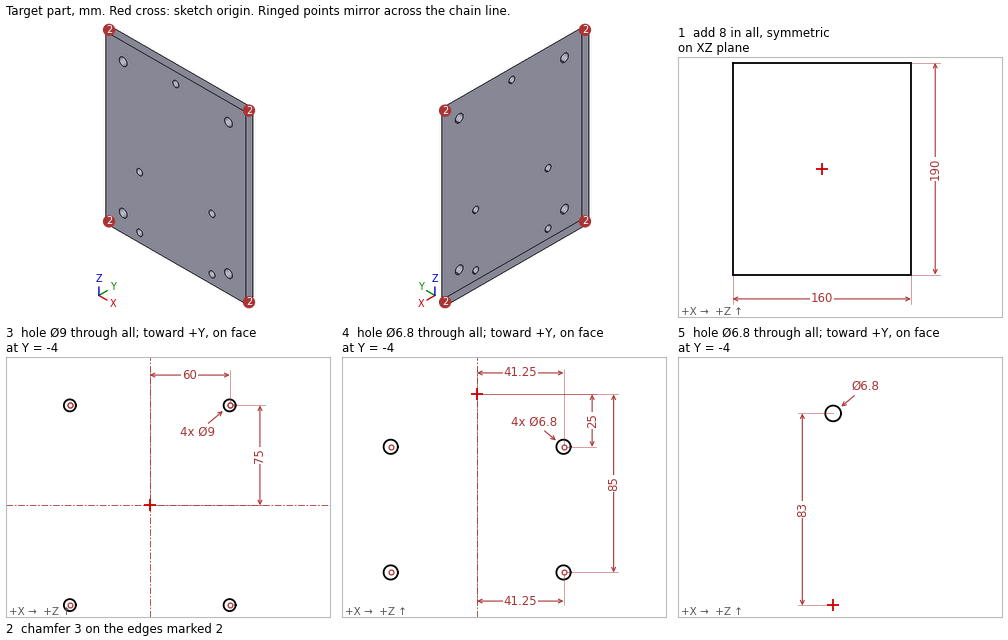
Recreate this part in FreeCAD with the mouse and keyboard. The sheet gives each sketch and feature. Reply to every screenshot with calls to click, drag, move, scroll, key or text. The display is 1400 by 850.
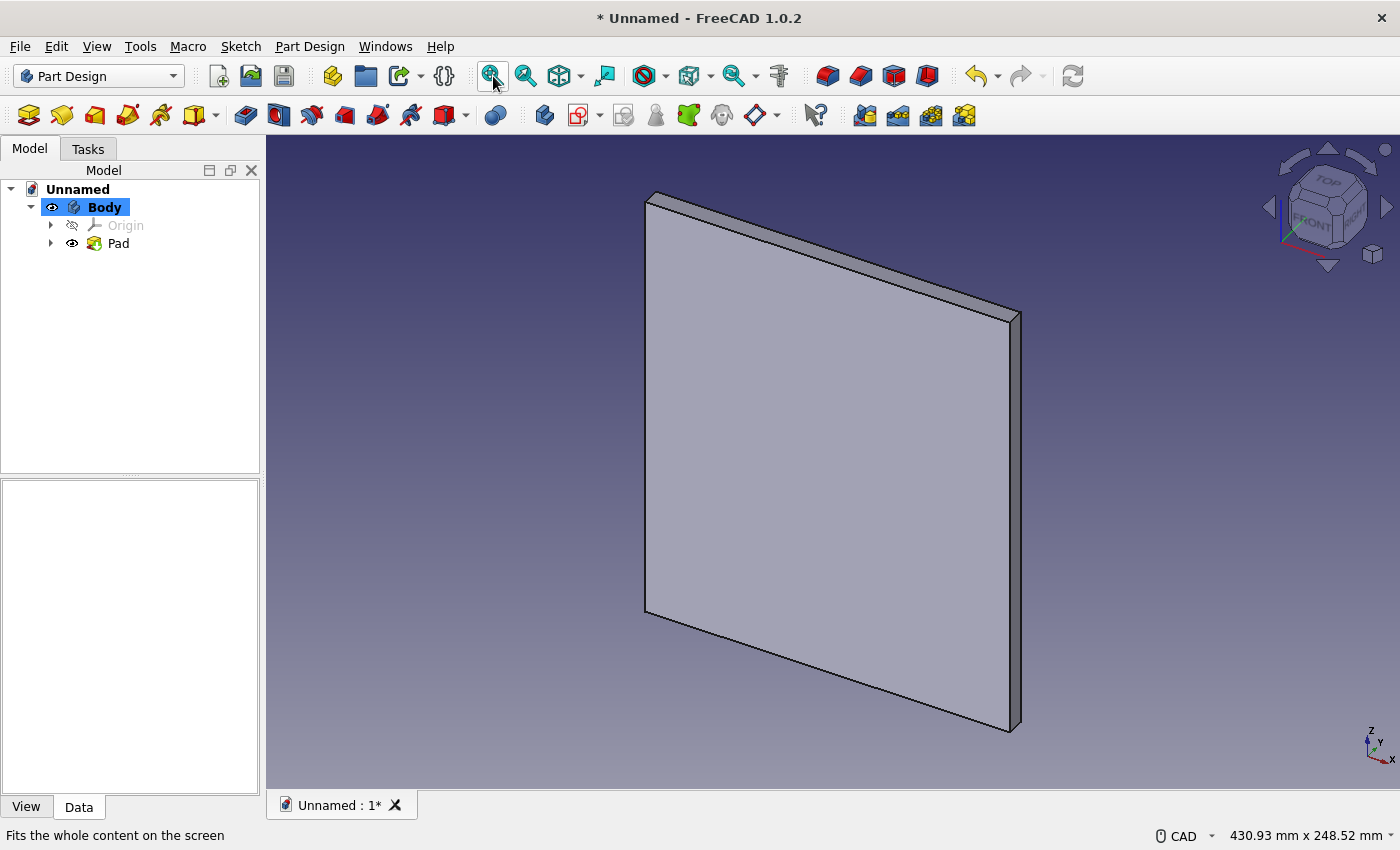
click(1015, 317)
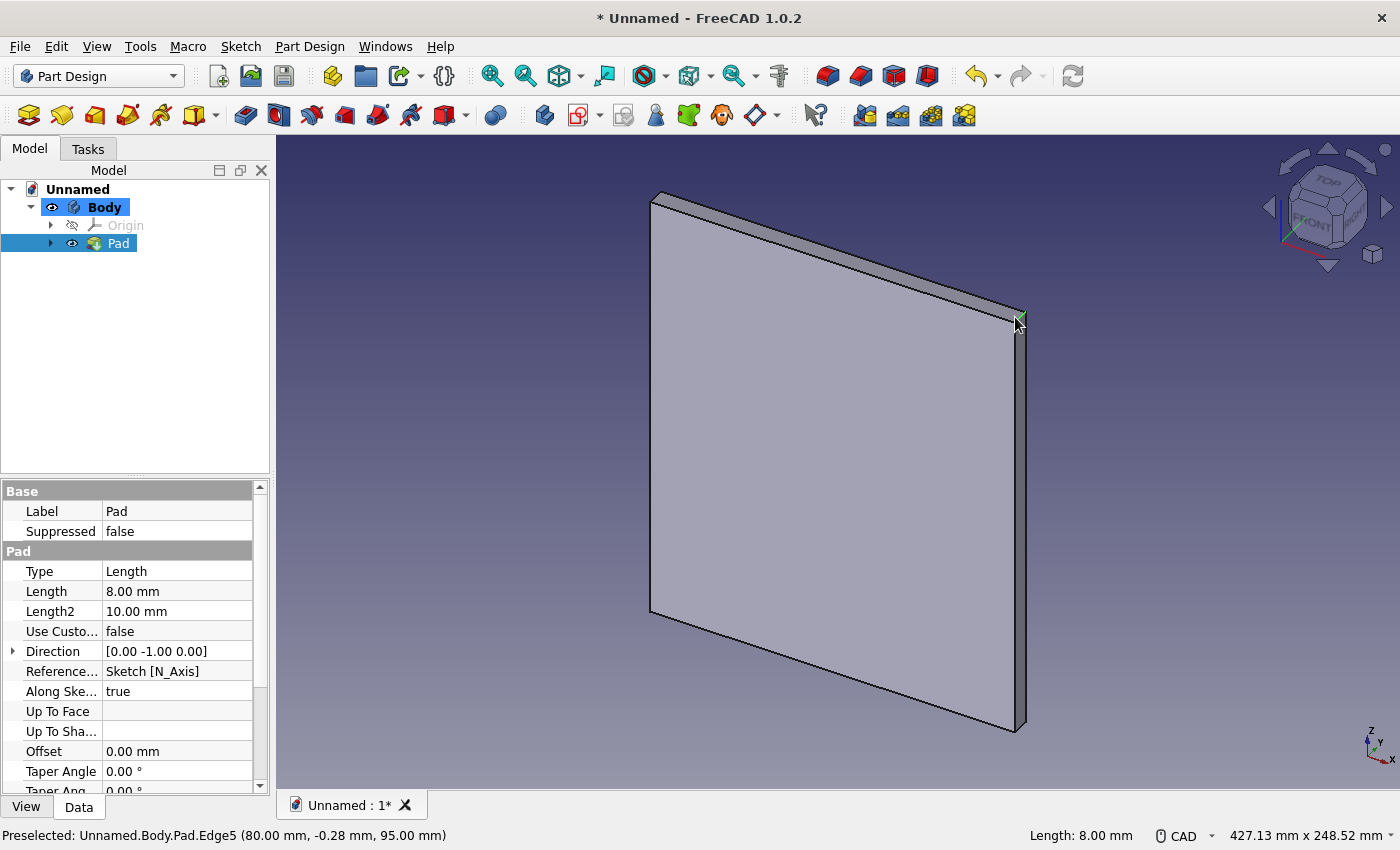
scroll(656, 196, up, 4)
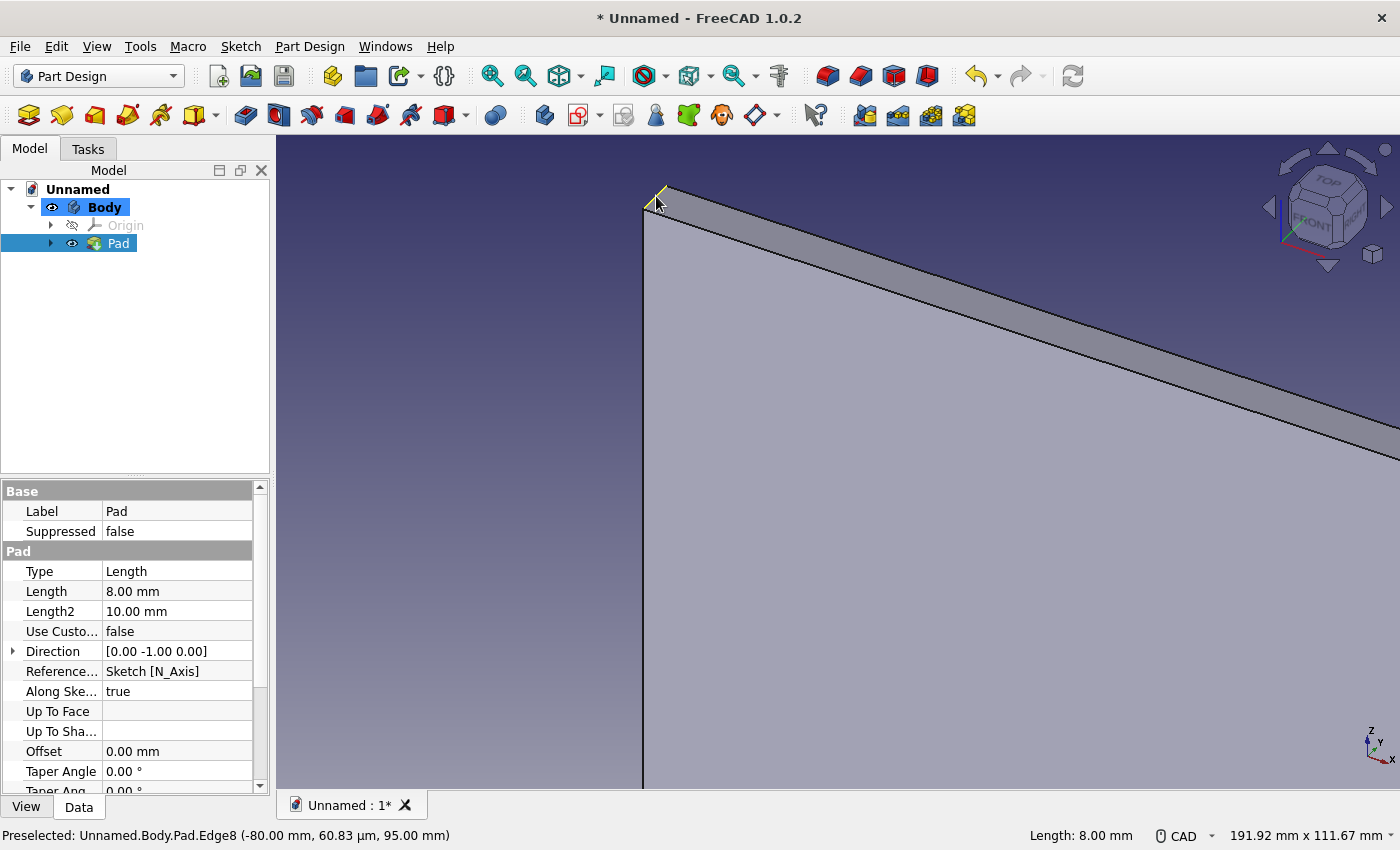
click(493, 76)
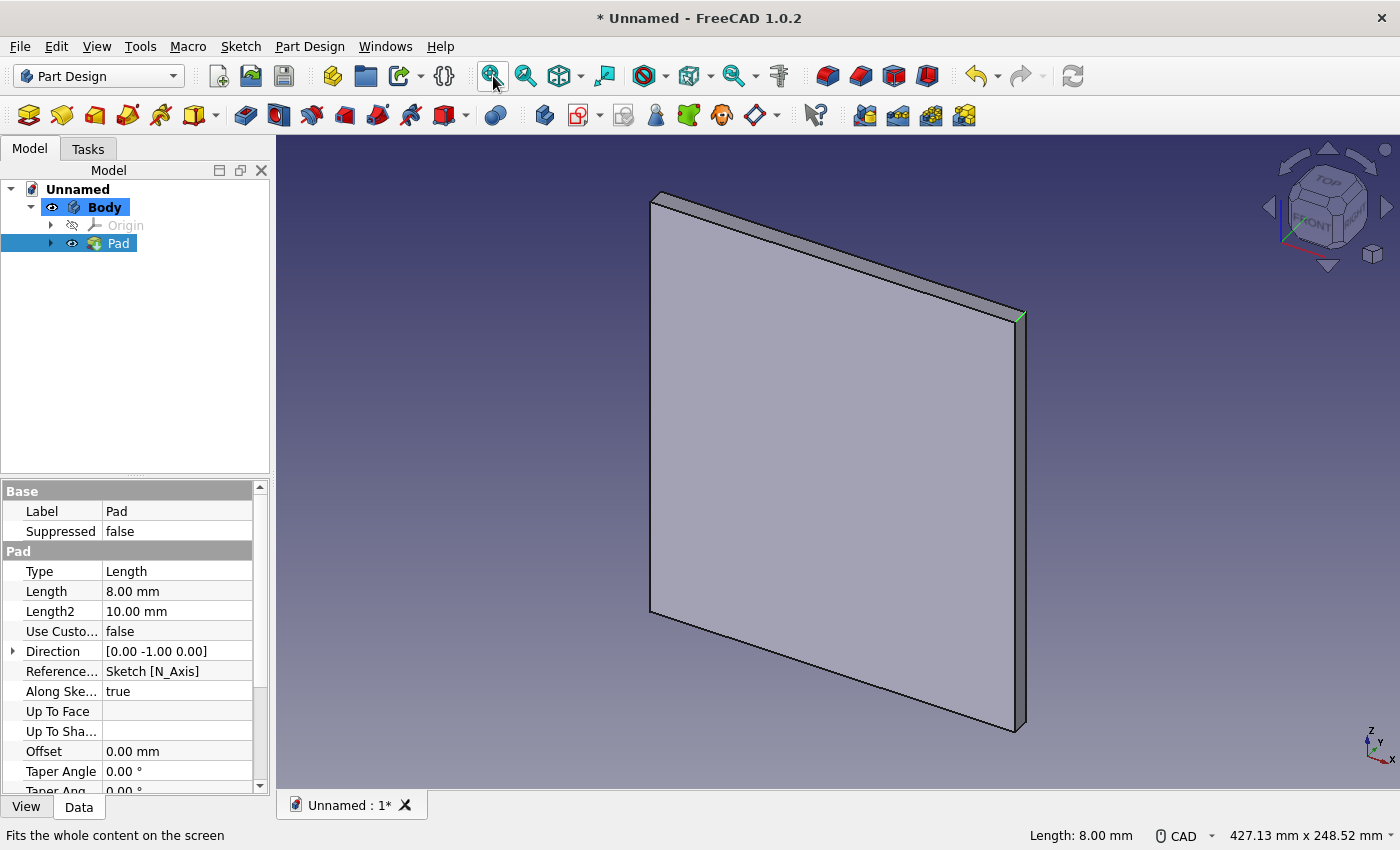
key(0)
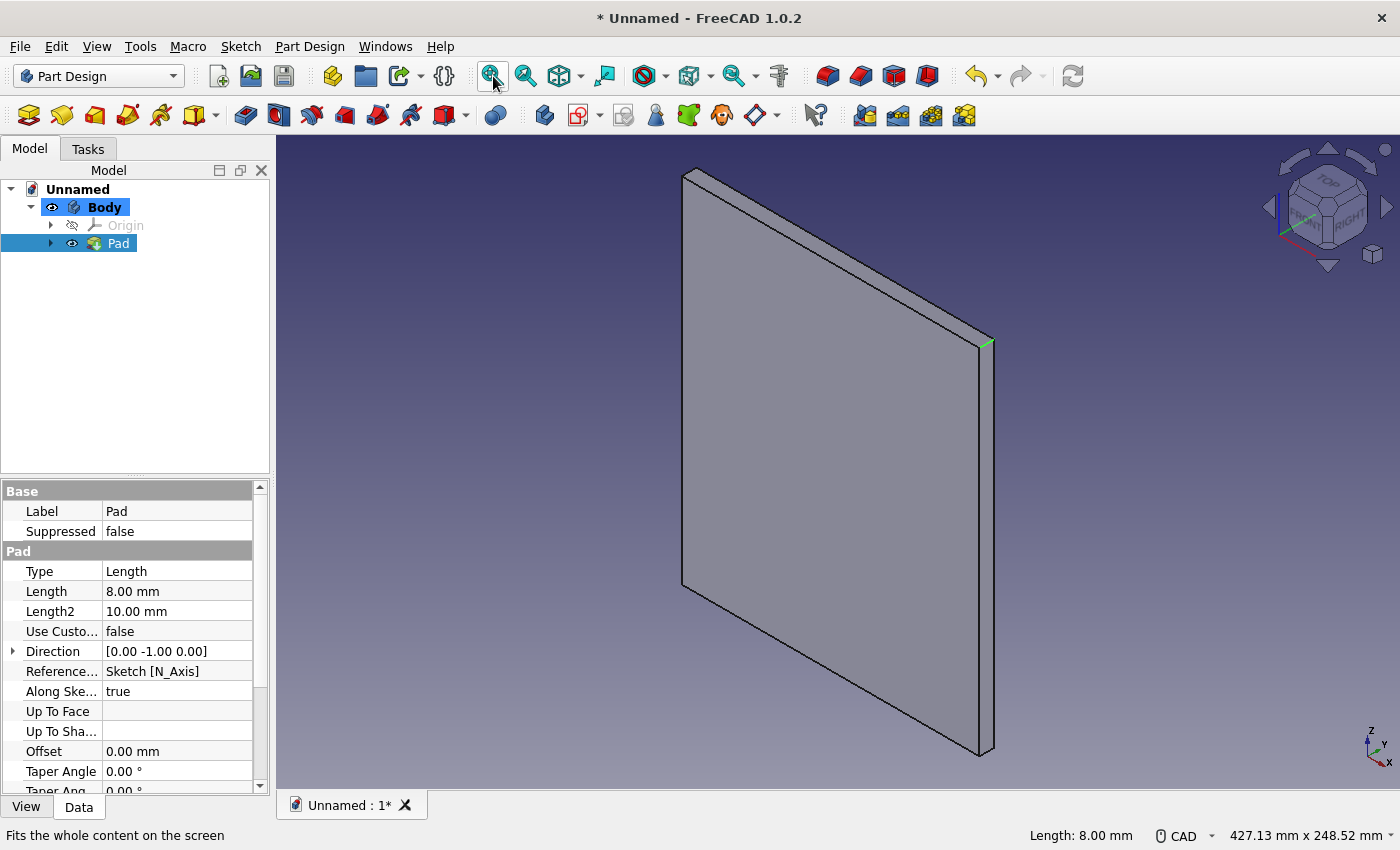
scroll(689, 171, up, 4)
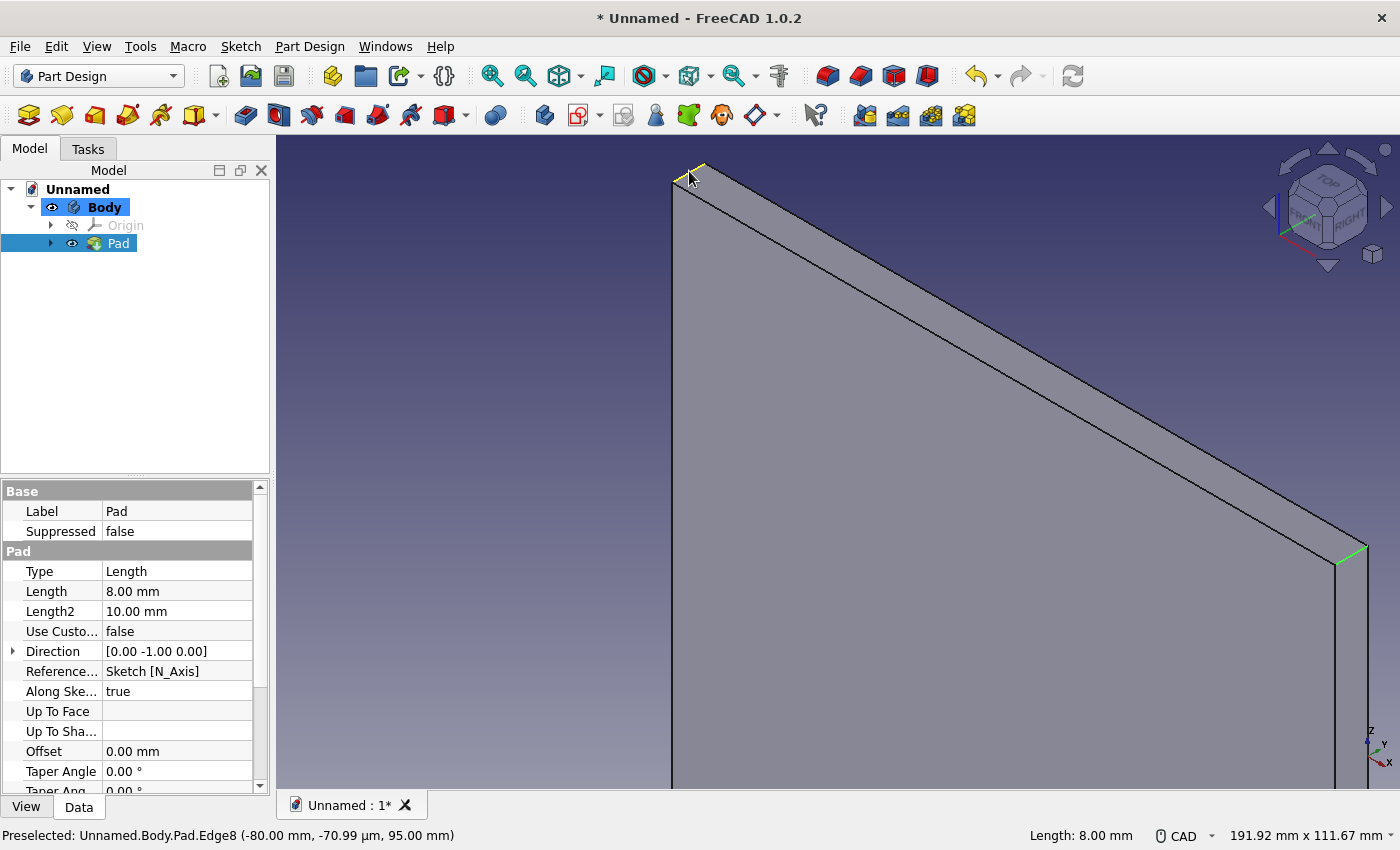
click(493, 76)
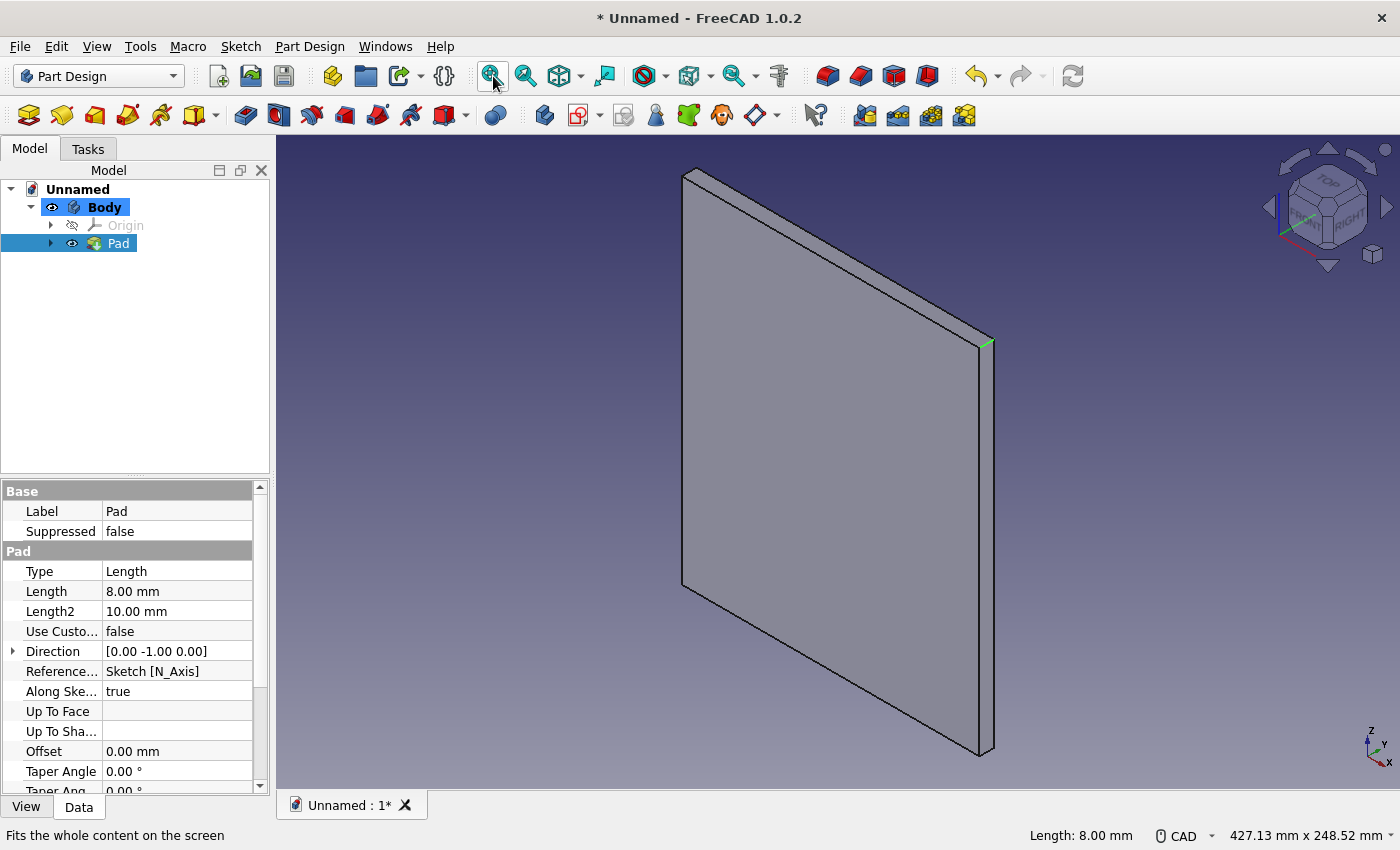
key(2)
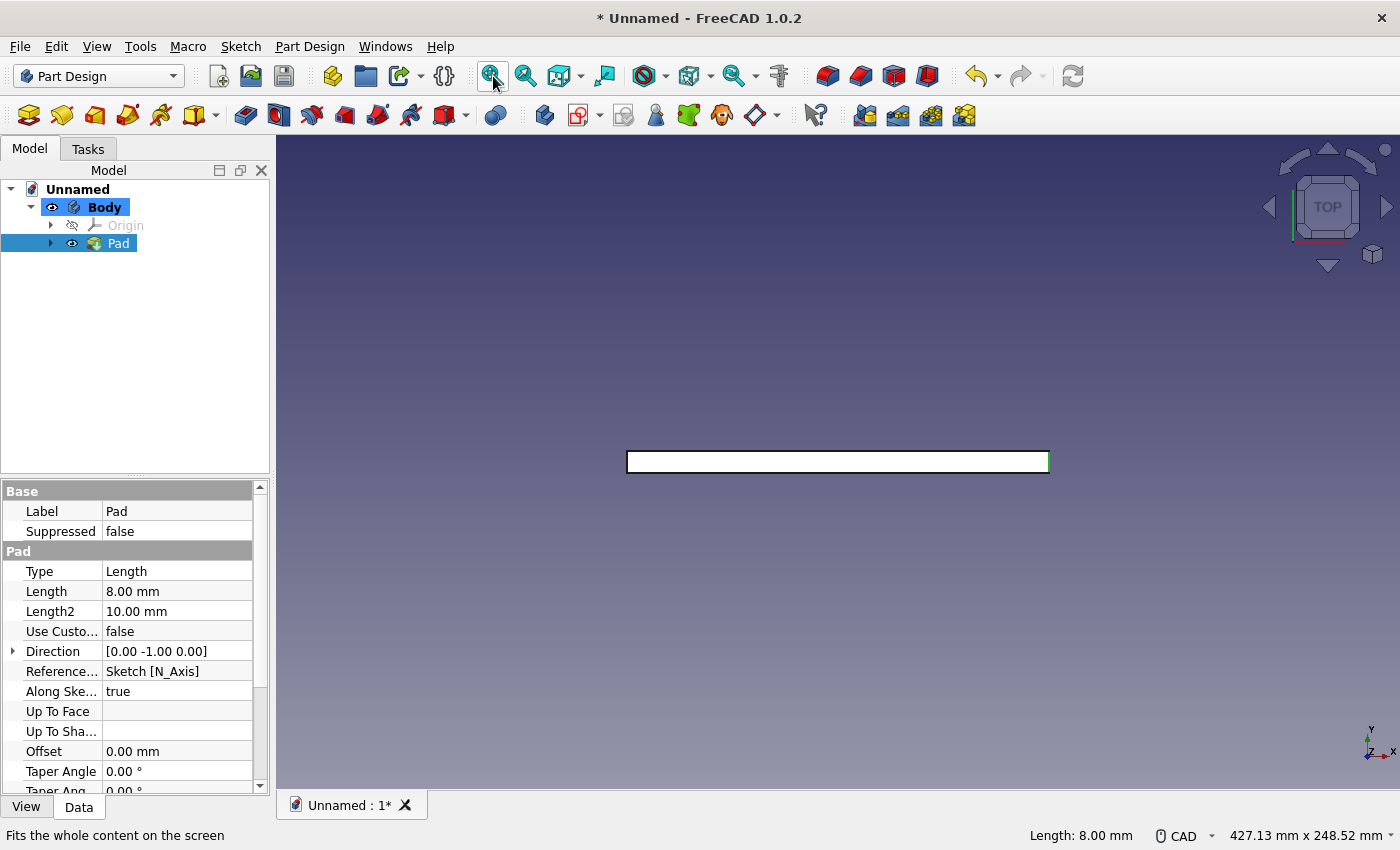
key(v)
key(f)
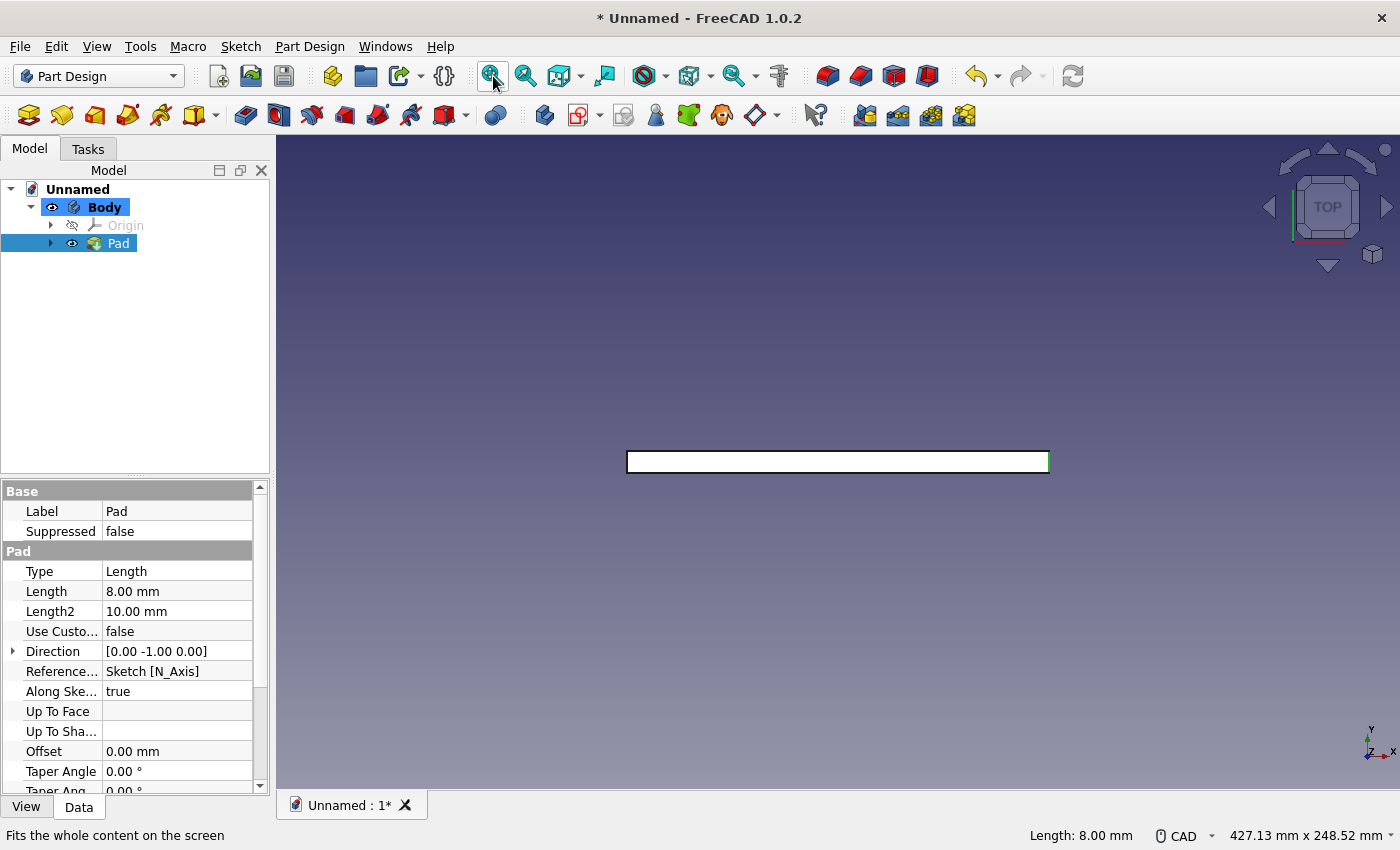
click(627, 461, ctrl)